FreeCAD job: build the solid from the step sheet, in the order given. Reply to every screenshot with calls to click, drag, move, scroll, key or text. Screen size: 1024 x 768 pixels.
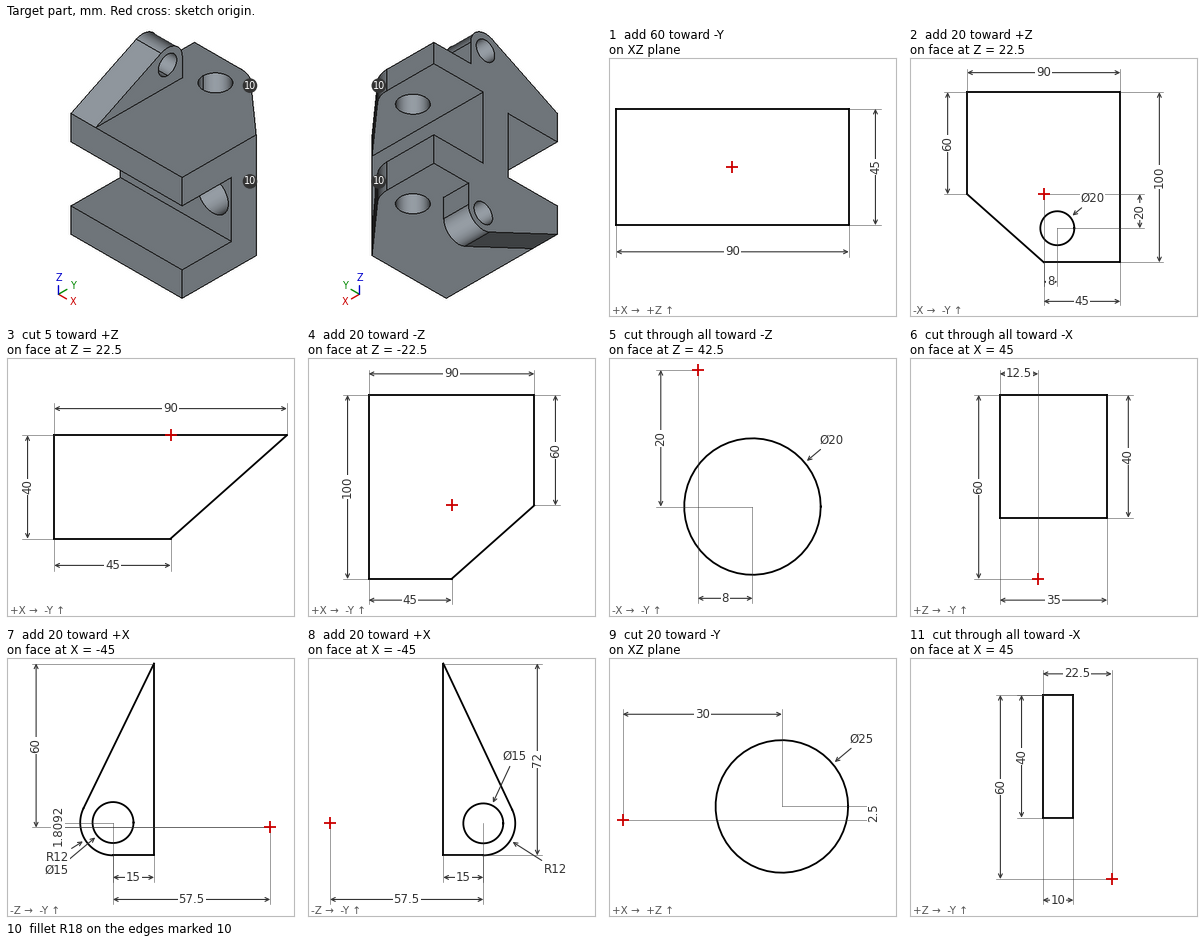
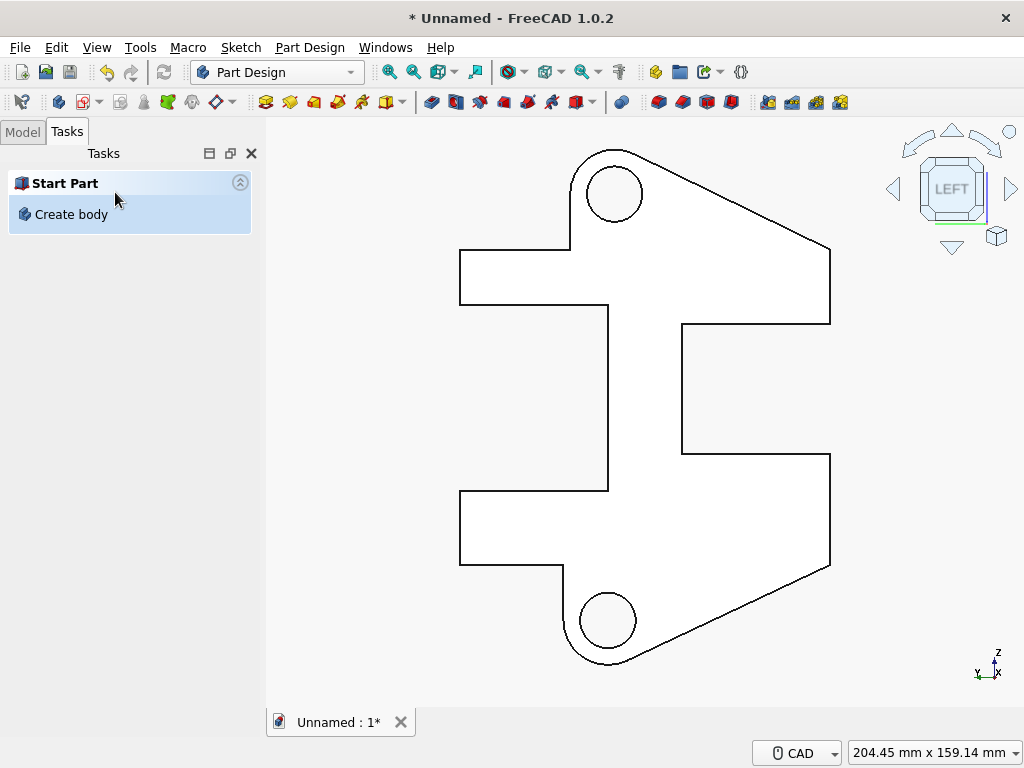
key(0)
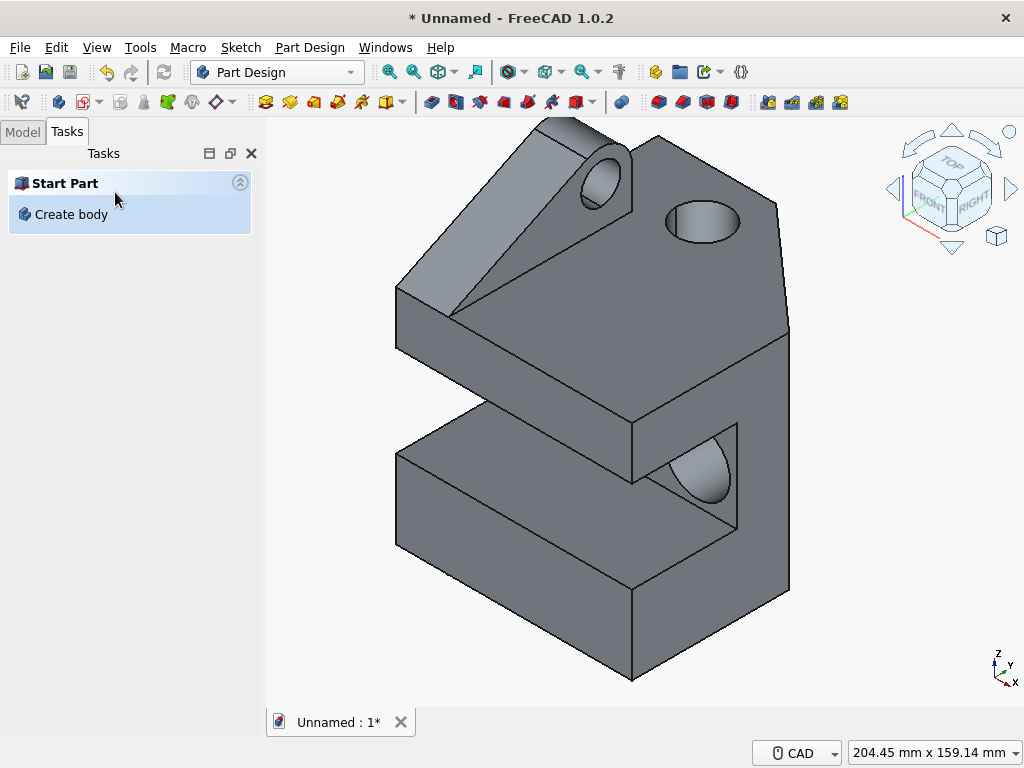
key(v)
key(f)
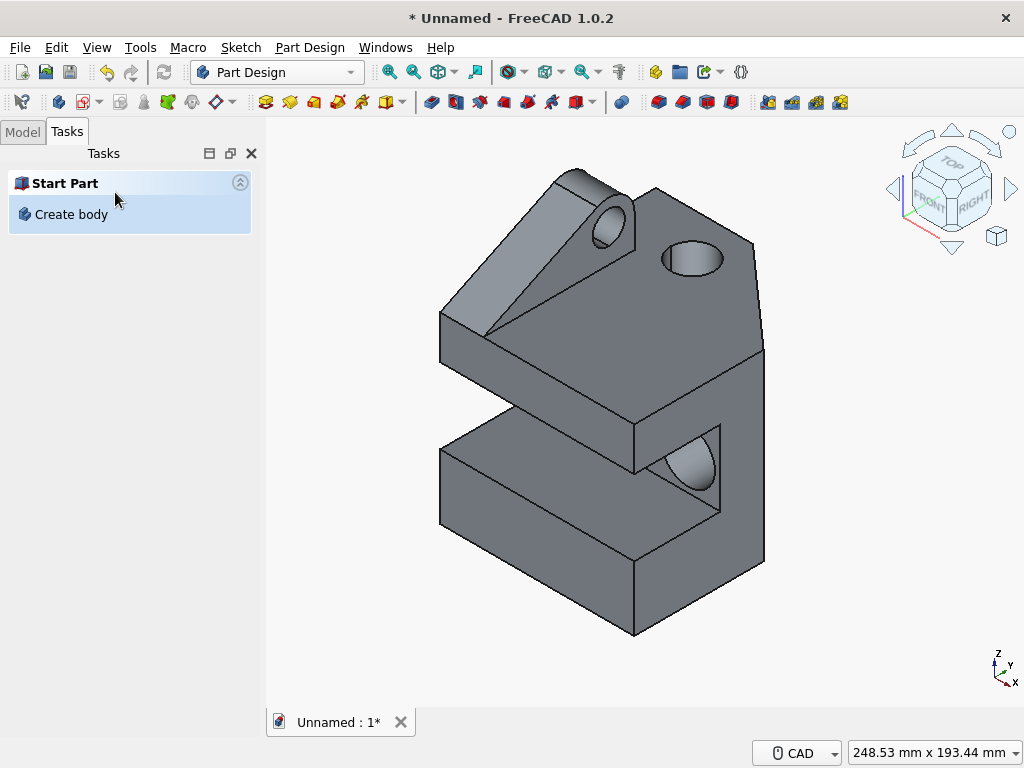
key(2)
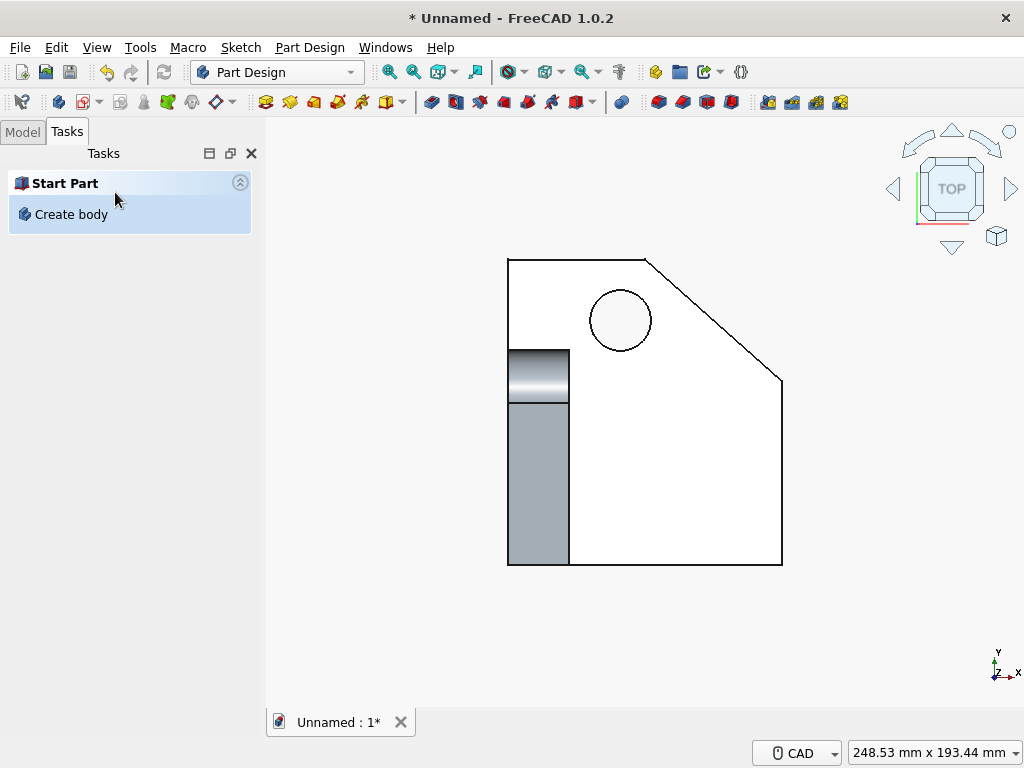
key(1)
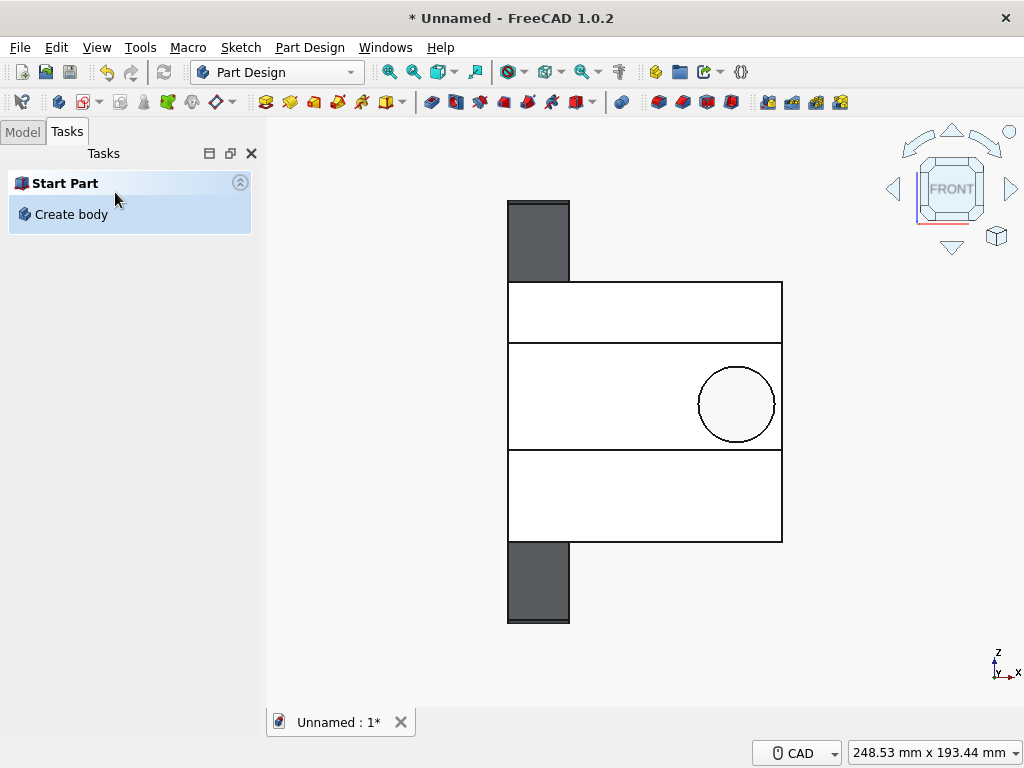
key(3)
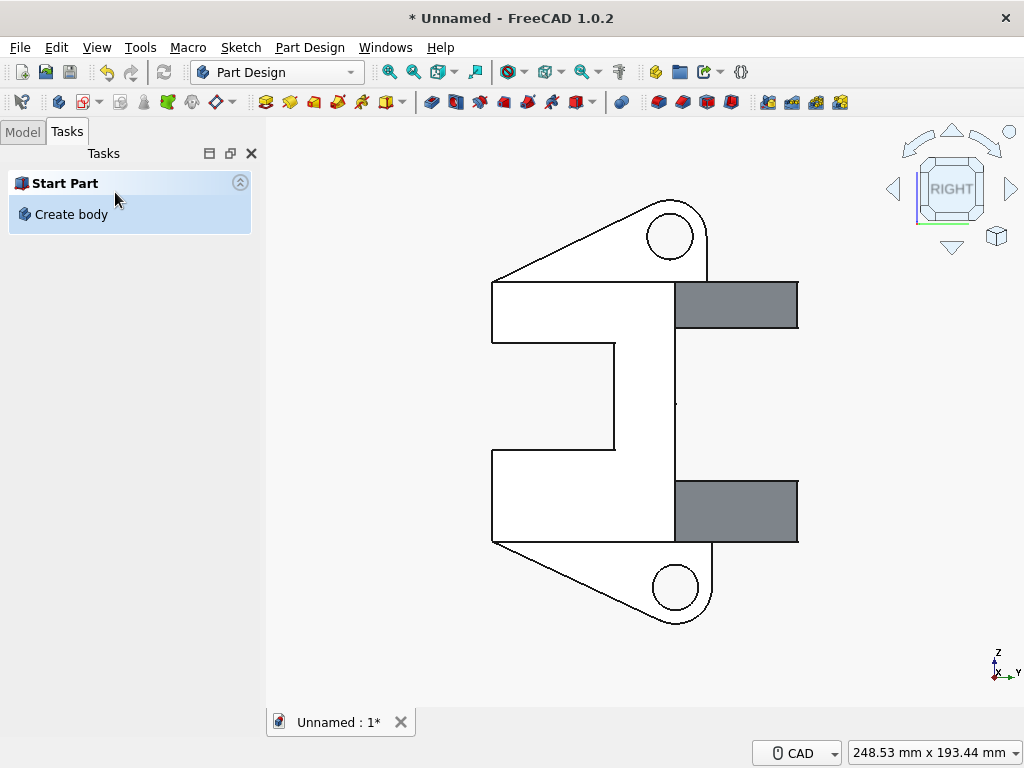
key(5)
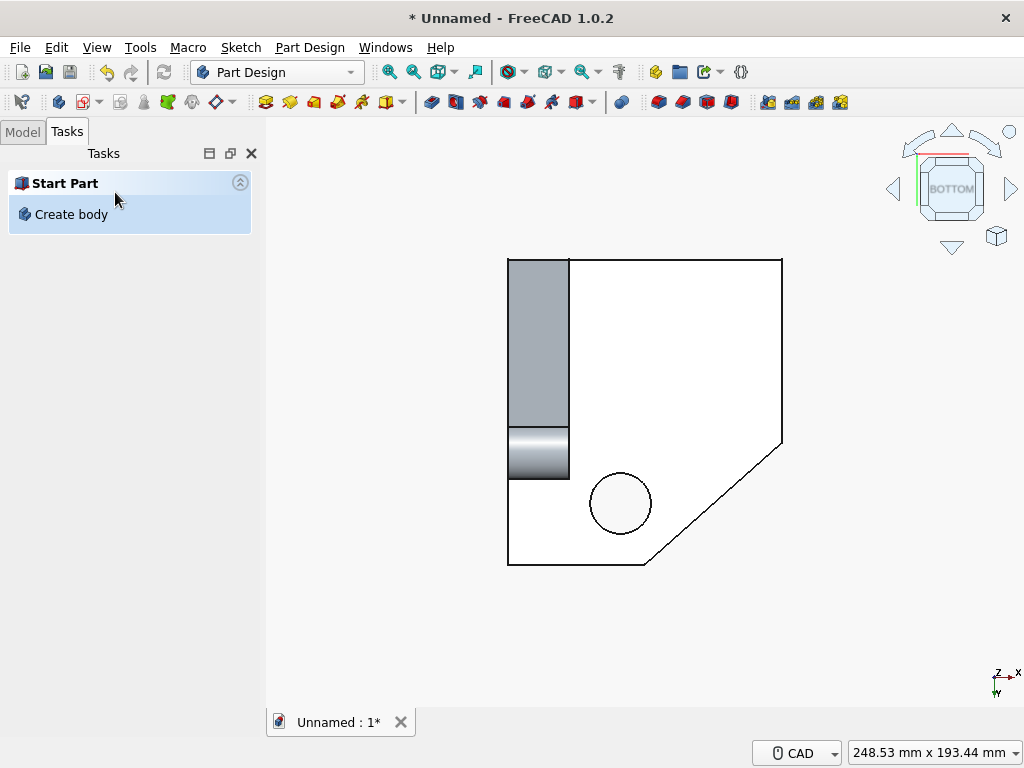
key(4)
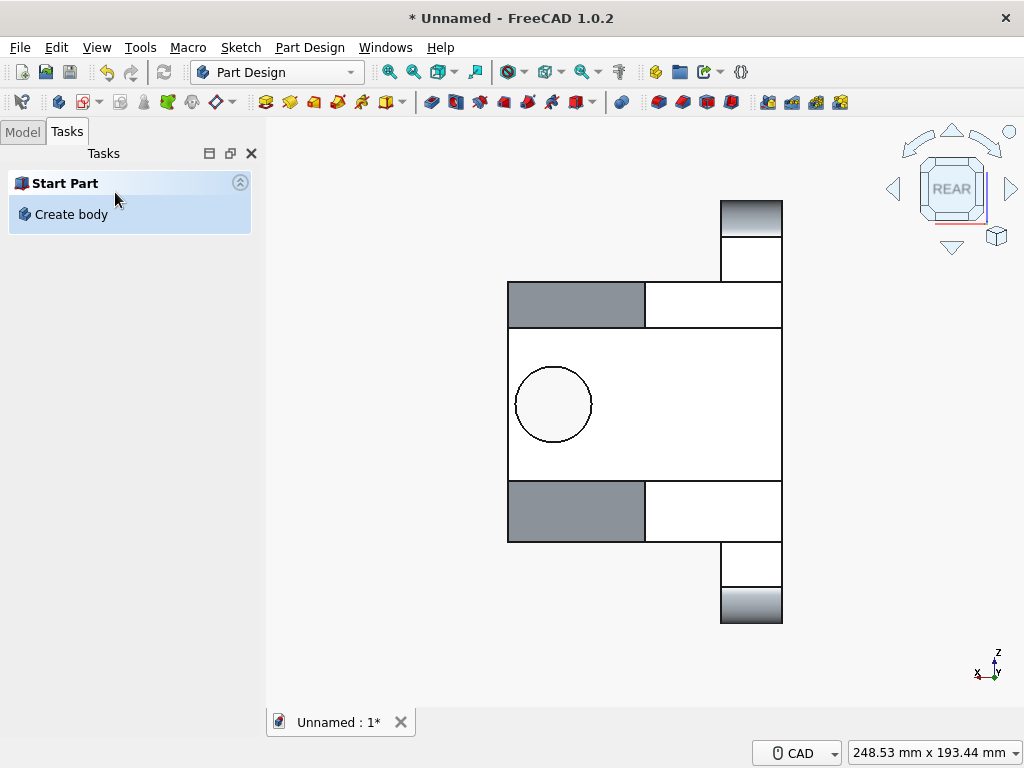
click(645, 304)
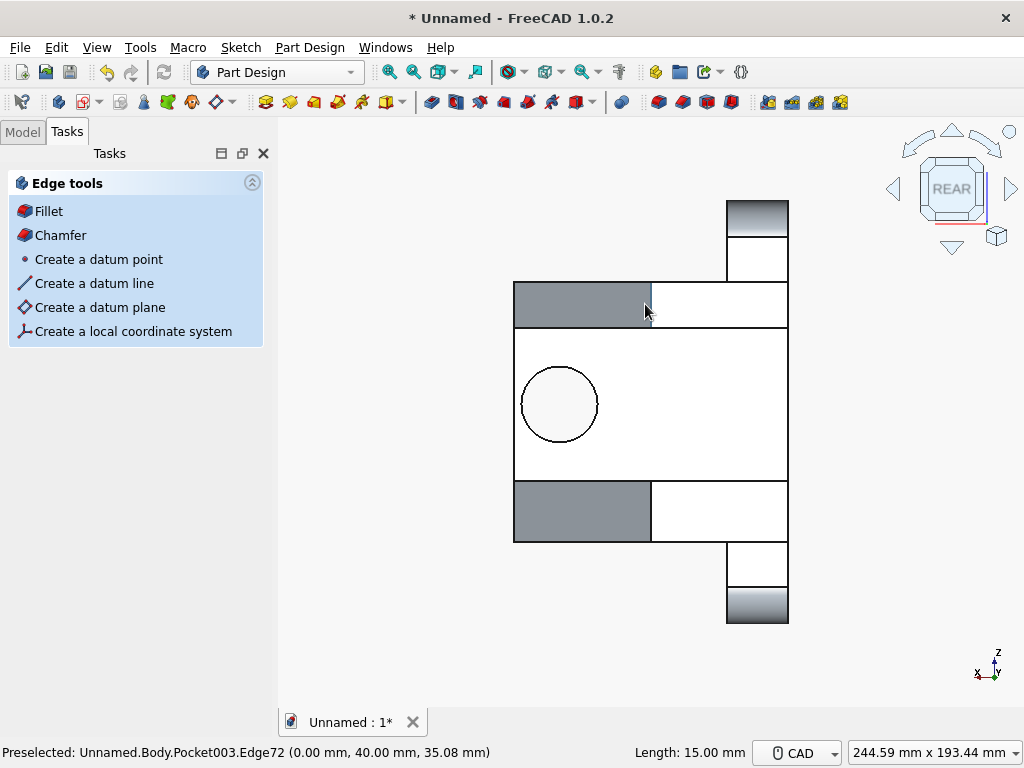
click(651, 510, ctrl)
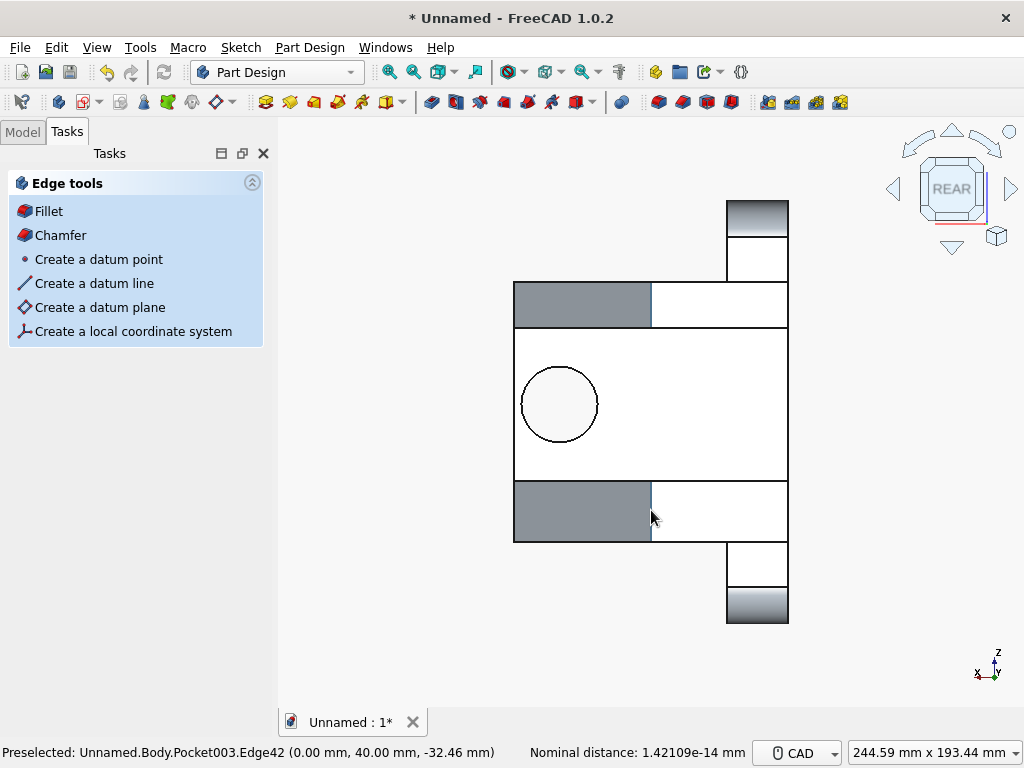
click(660, 102)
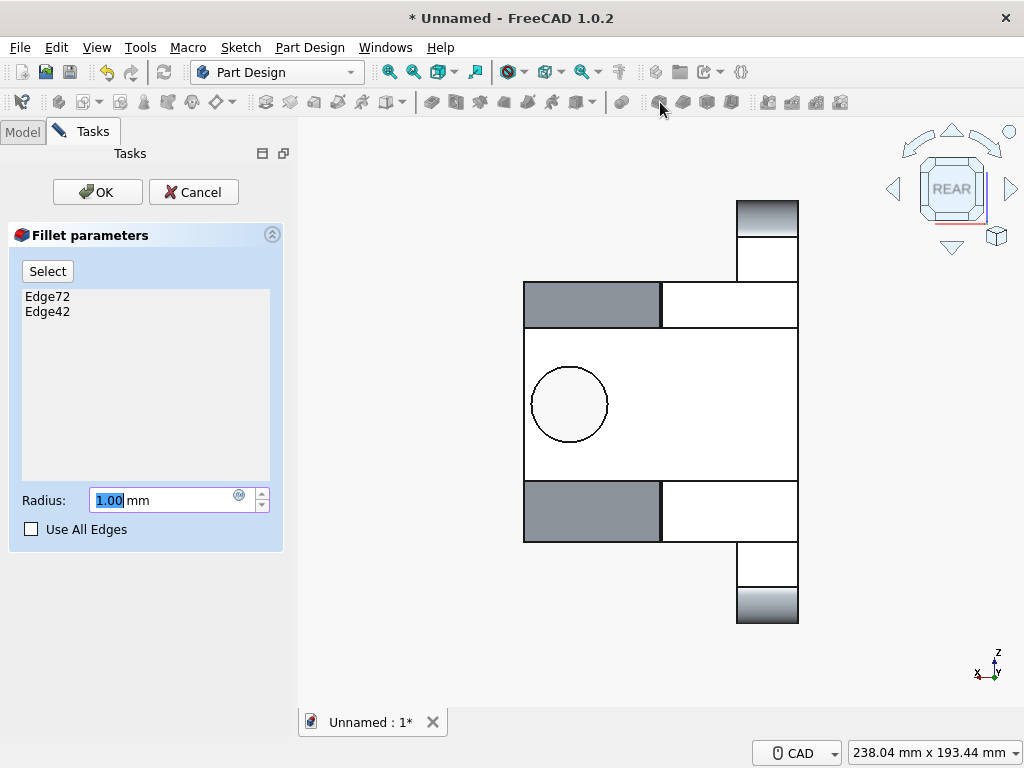
text(18)
key(Tab)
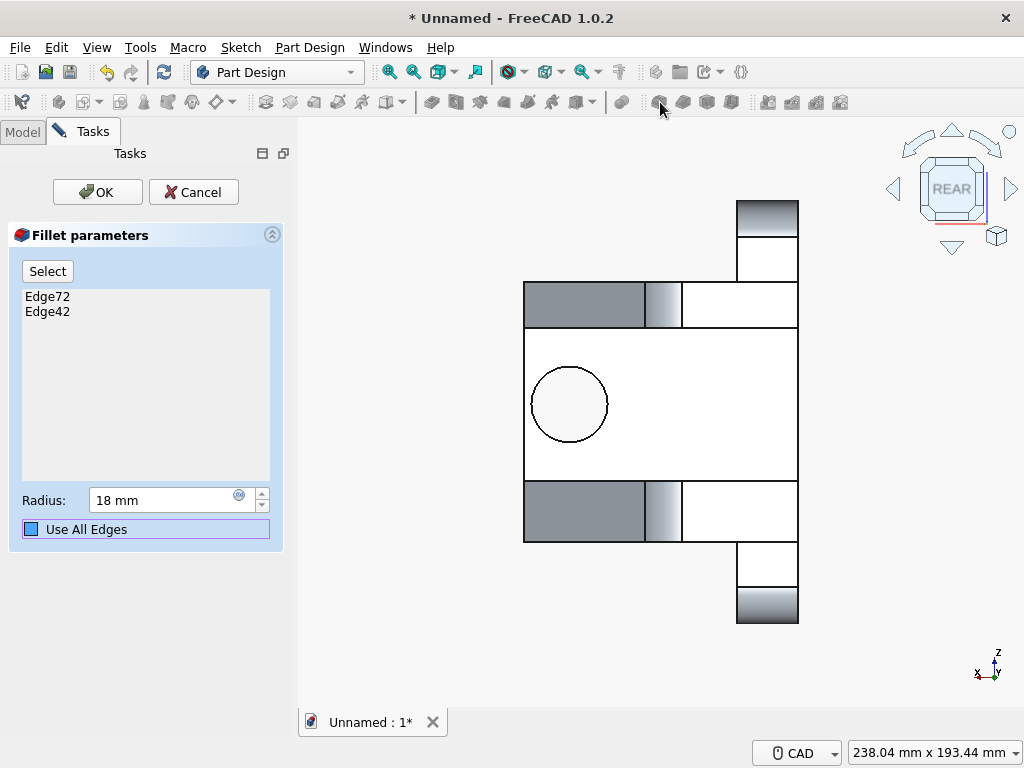
click(98, 192)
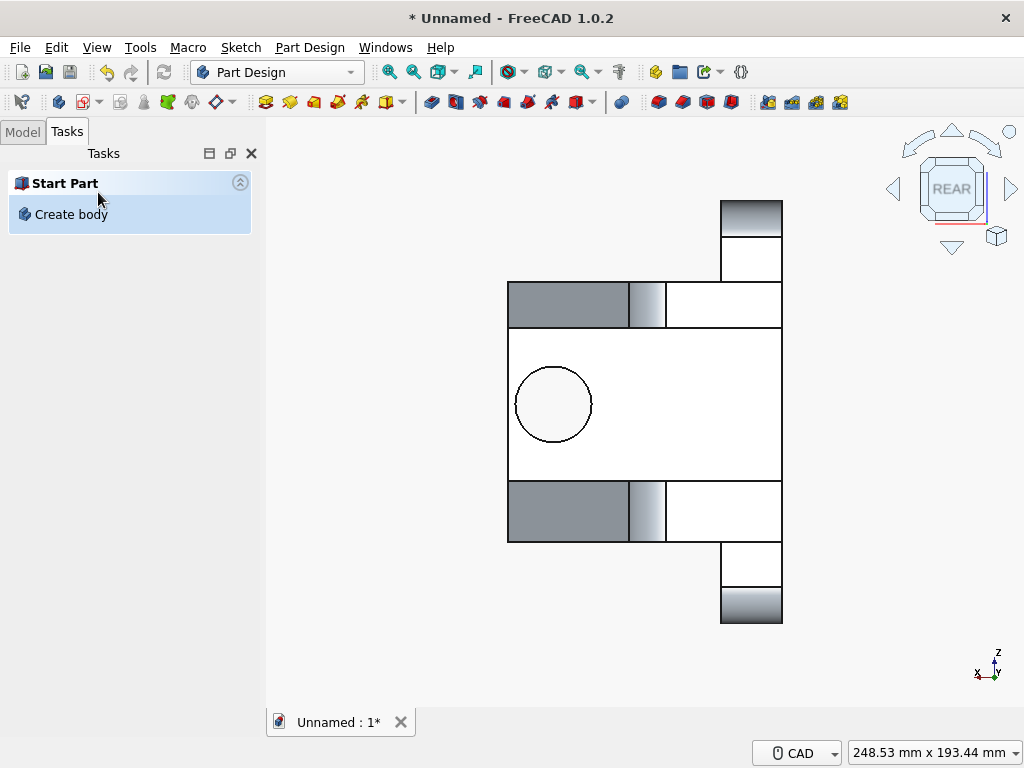
key(0)